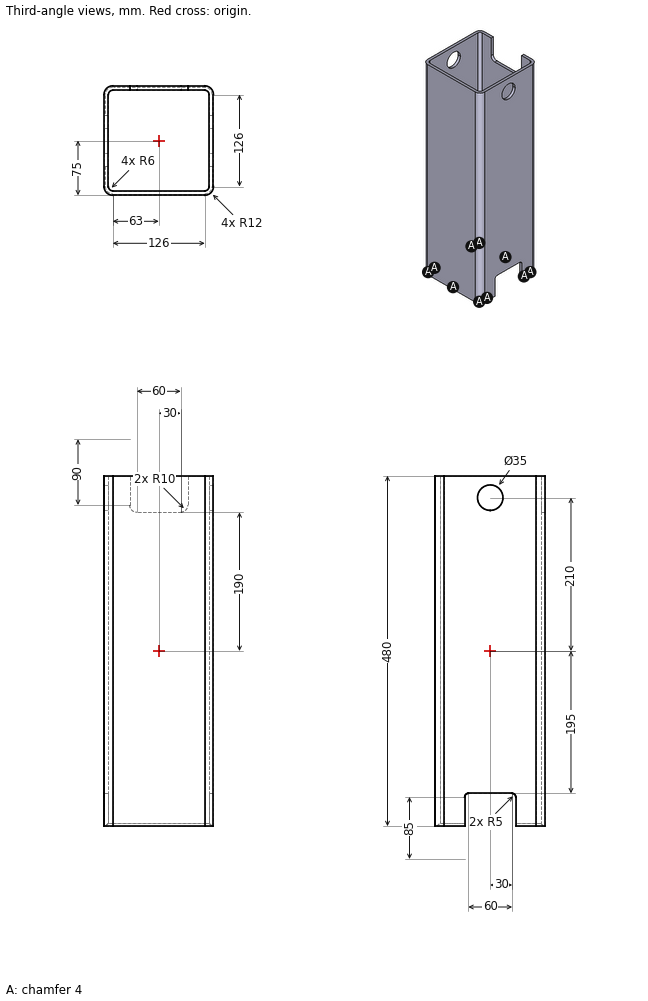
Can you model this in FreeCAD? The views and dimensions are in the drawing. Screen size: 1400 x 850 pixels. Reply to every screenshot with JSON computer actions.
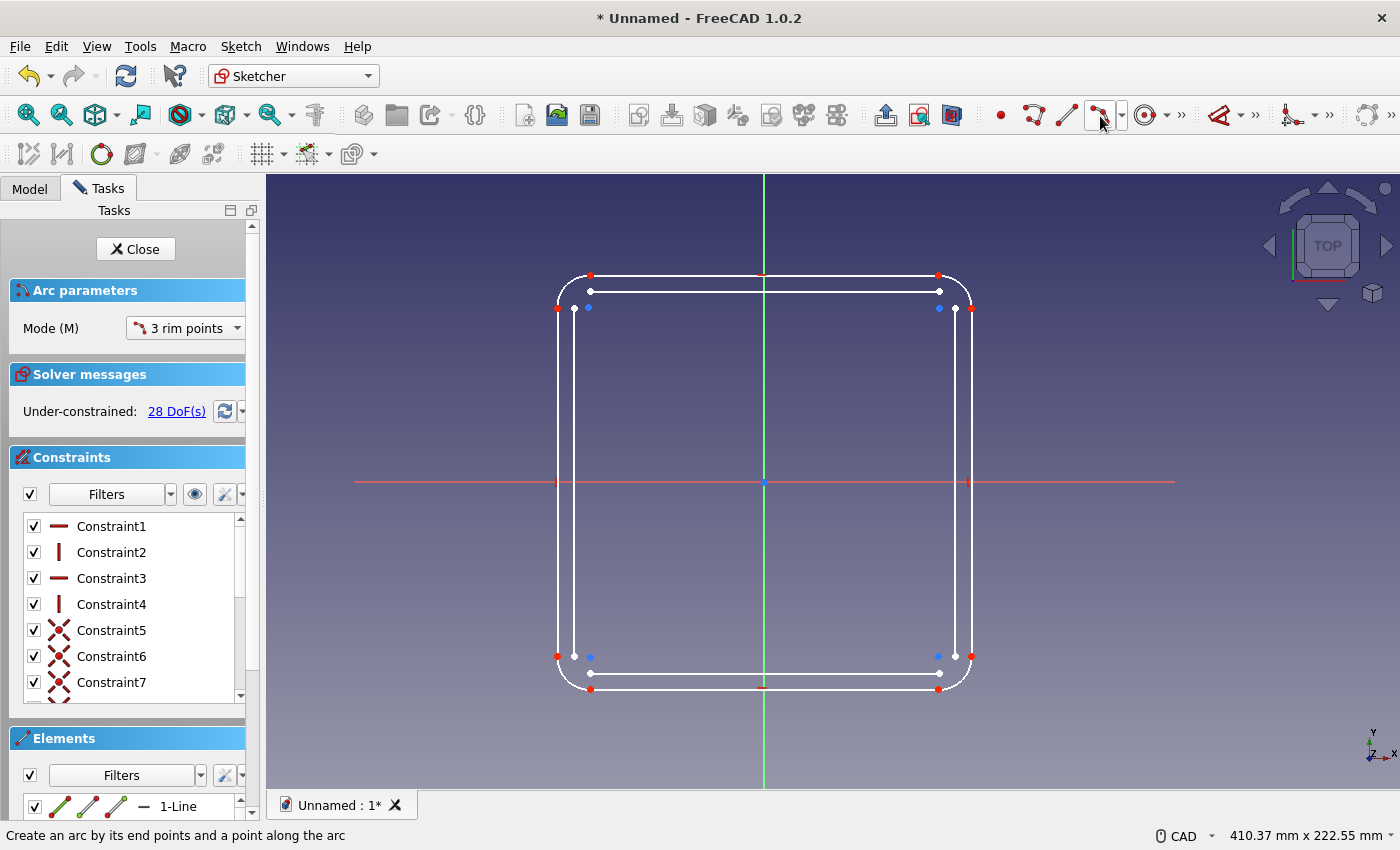
{"action": "left_click", "coordinate": [590, 674]}
{"action": "left_click", "coordinate": [574, 657]}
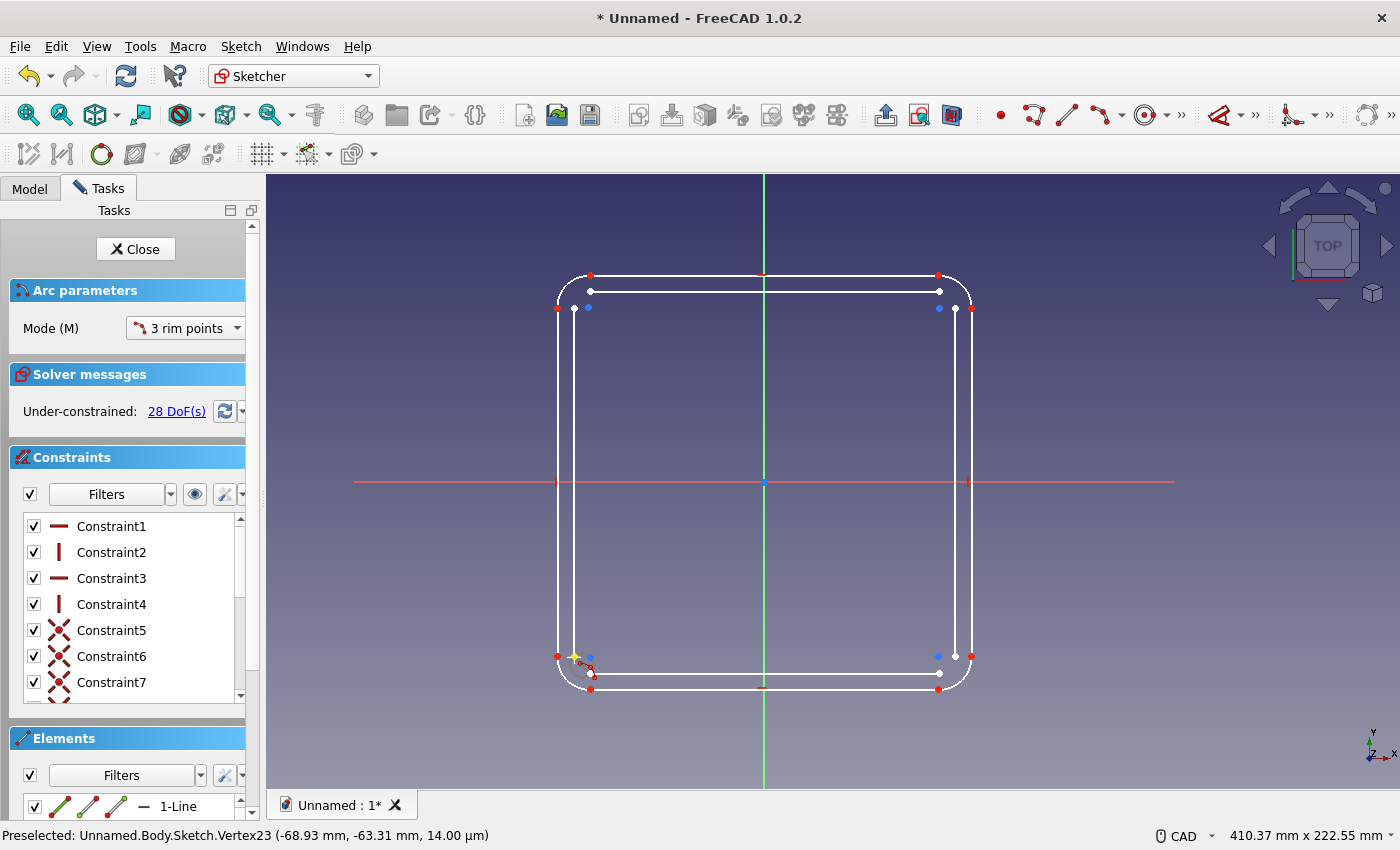
{"action": "scroll", "coordinate": [579, 668], "scroll_direction": "up", "scroll_amount": 6}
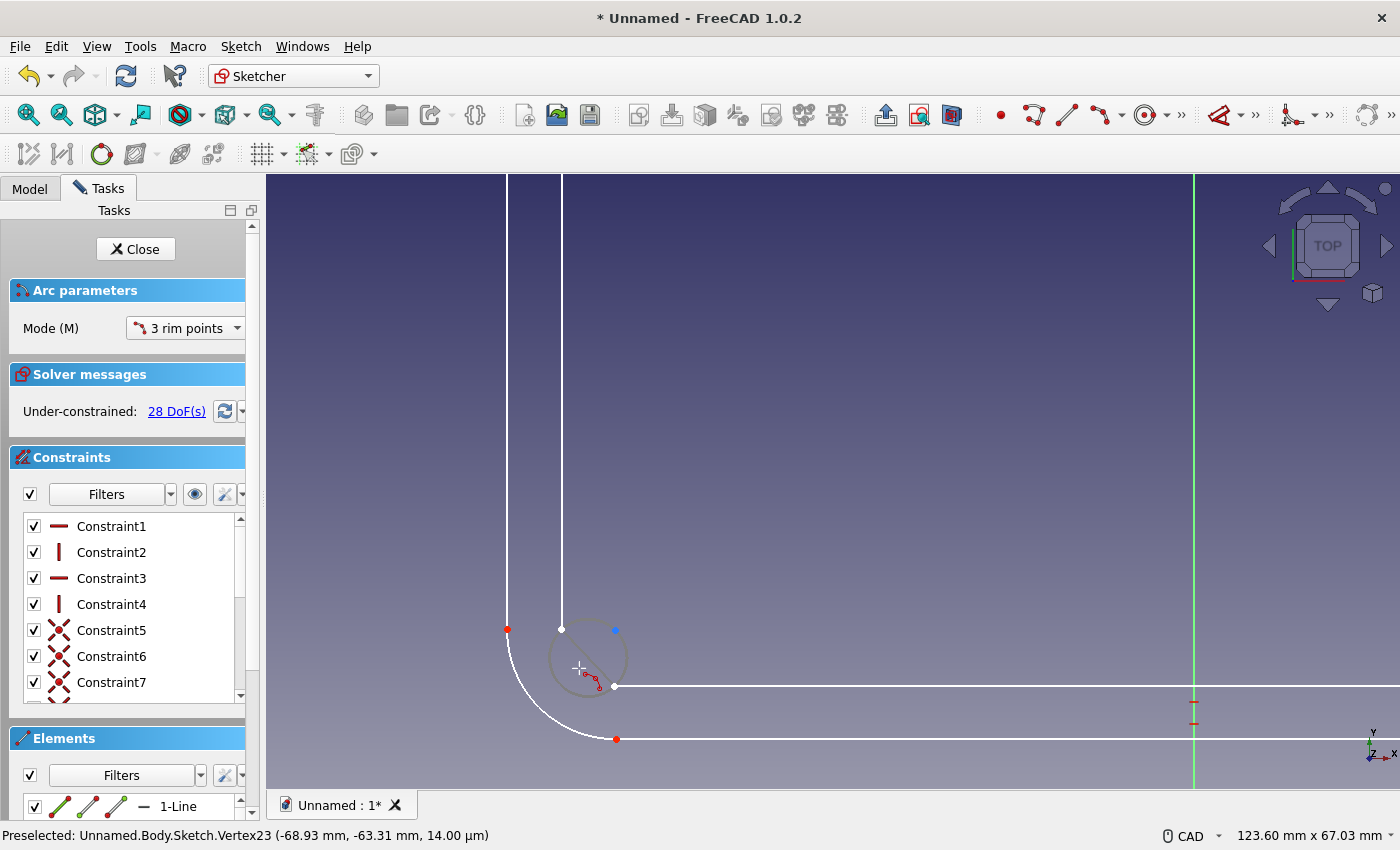
{"action": "left_click", "coordinate": [577, 666]}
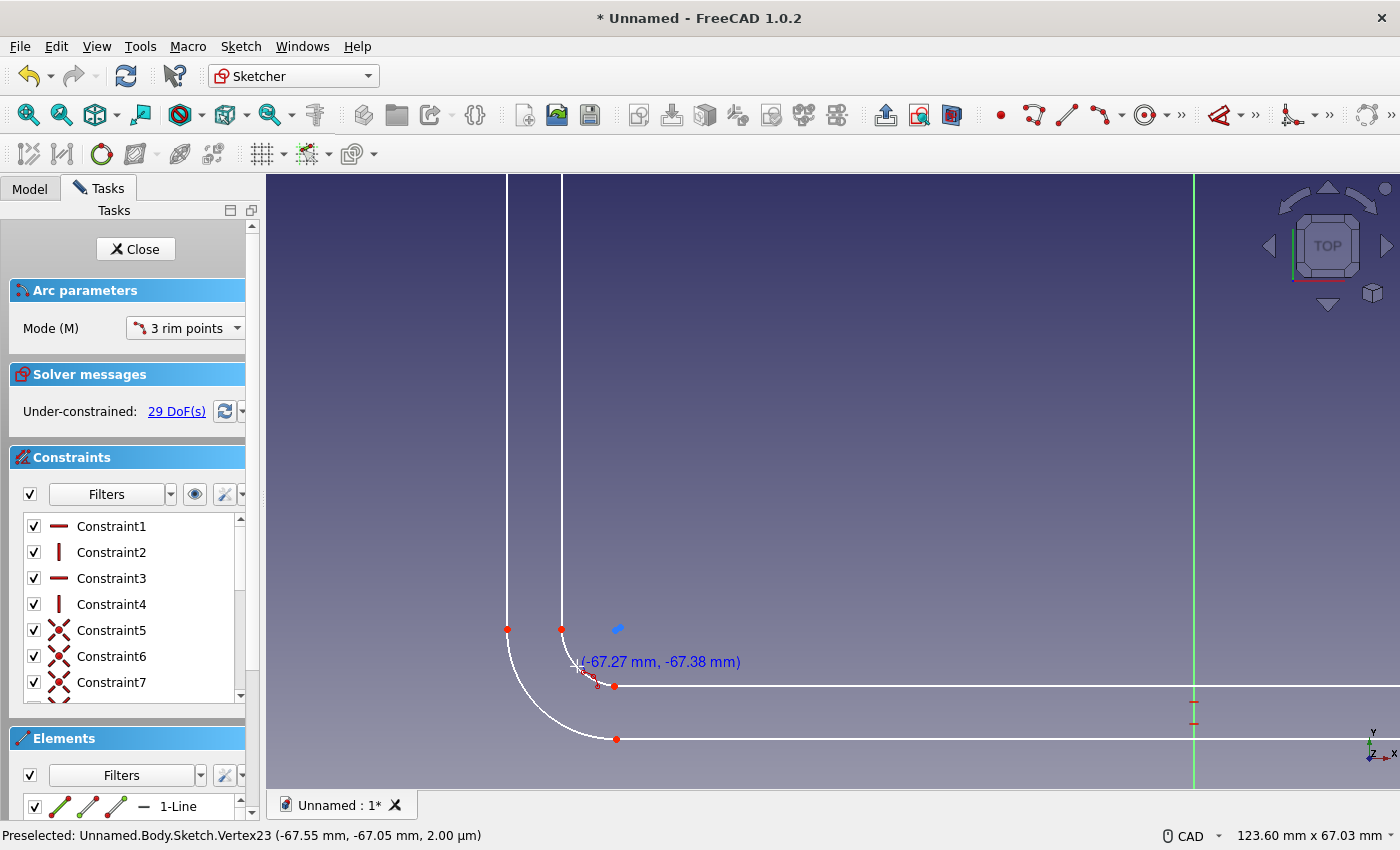
{"action": "scroll", "coordinate": [579, 668], "scroll_direction": "down", "scroll_amount": 6}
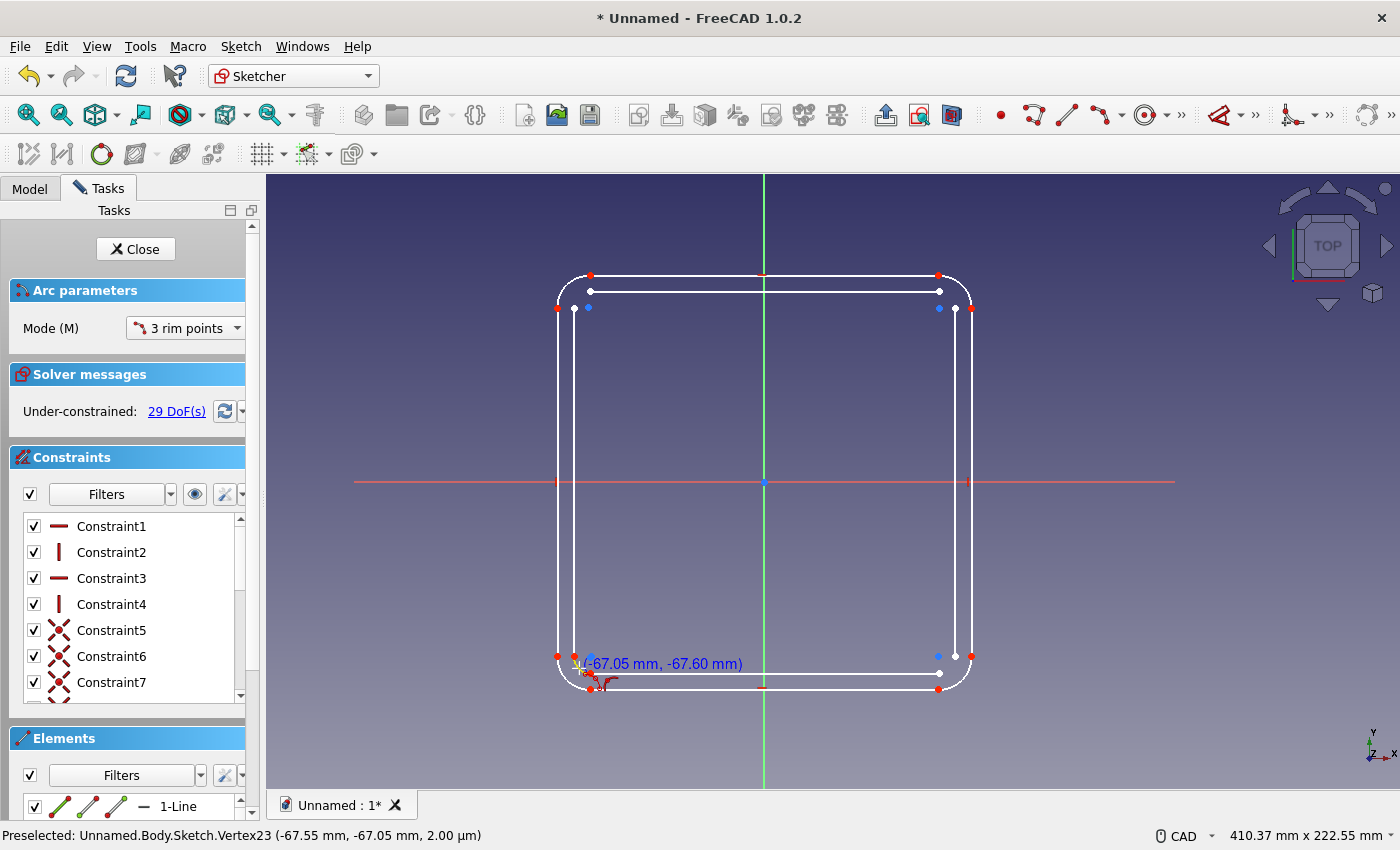
{"action": "left_click", "coordinate": [574, 309]}
{"action": "left_click", "coordinate": [590, 292]}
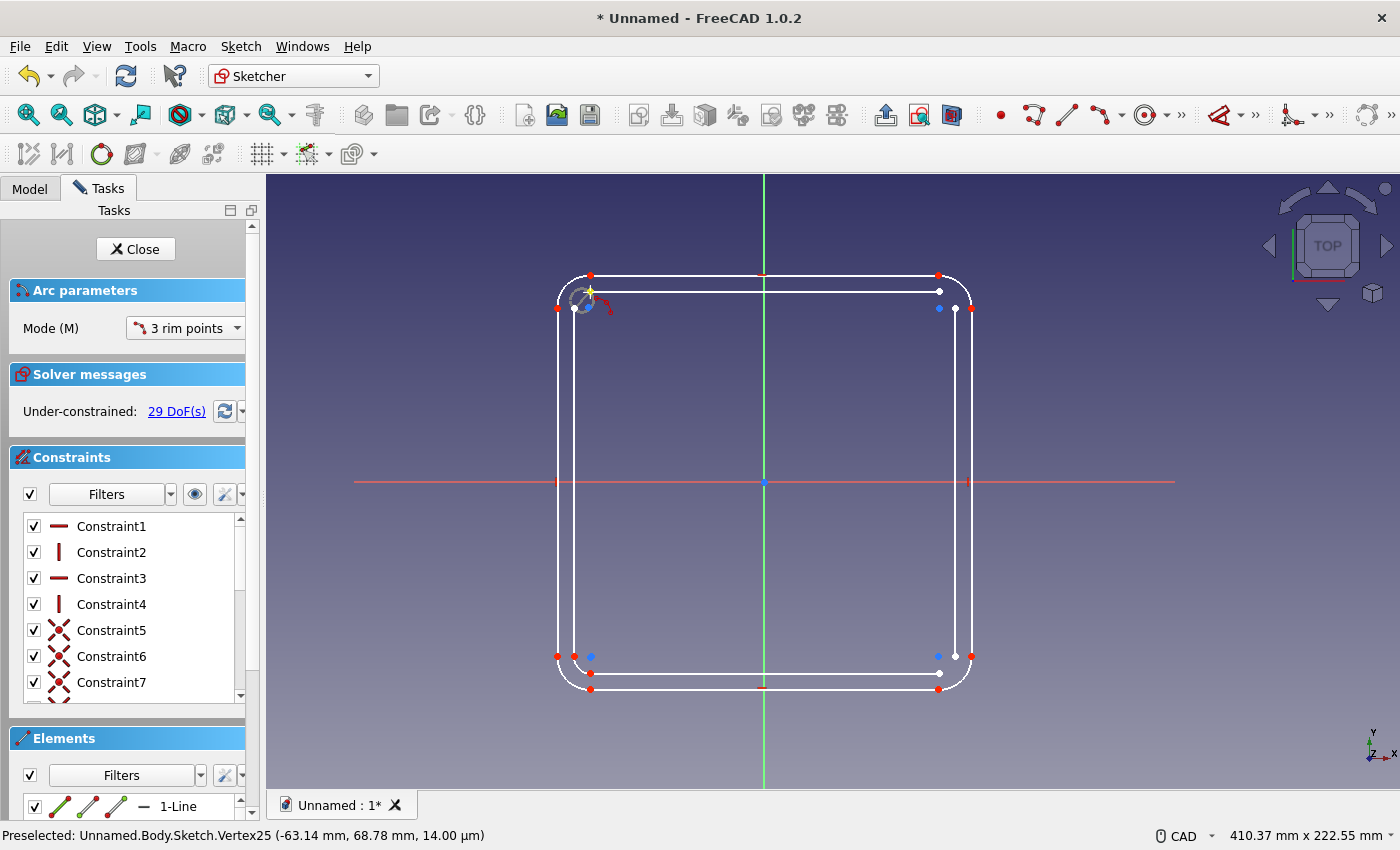
{"action": "scroll", "coordinate": [579, 296], "scroll_direction": "up", "scroll_amount": 6}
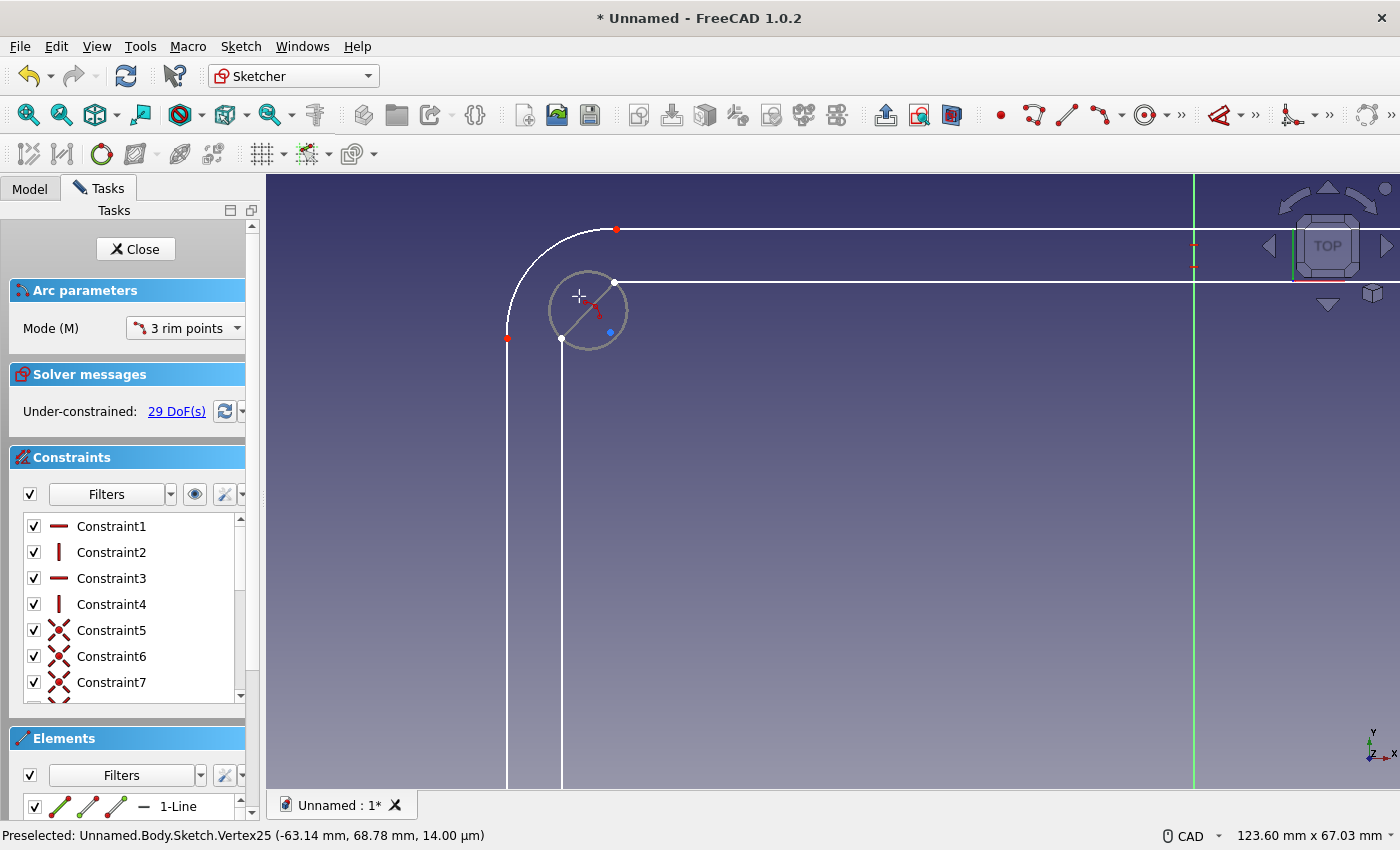
{"action": "left_click", "coordinate": [577, 296]}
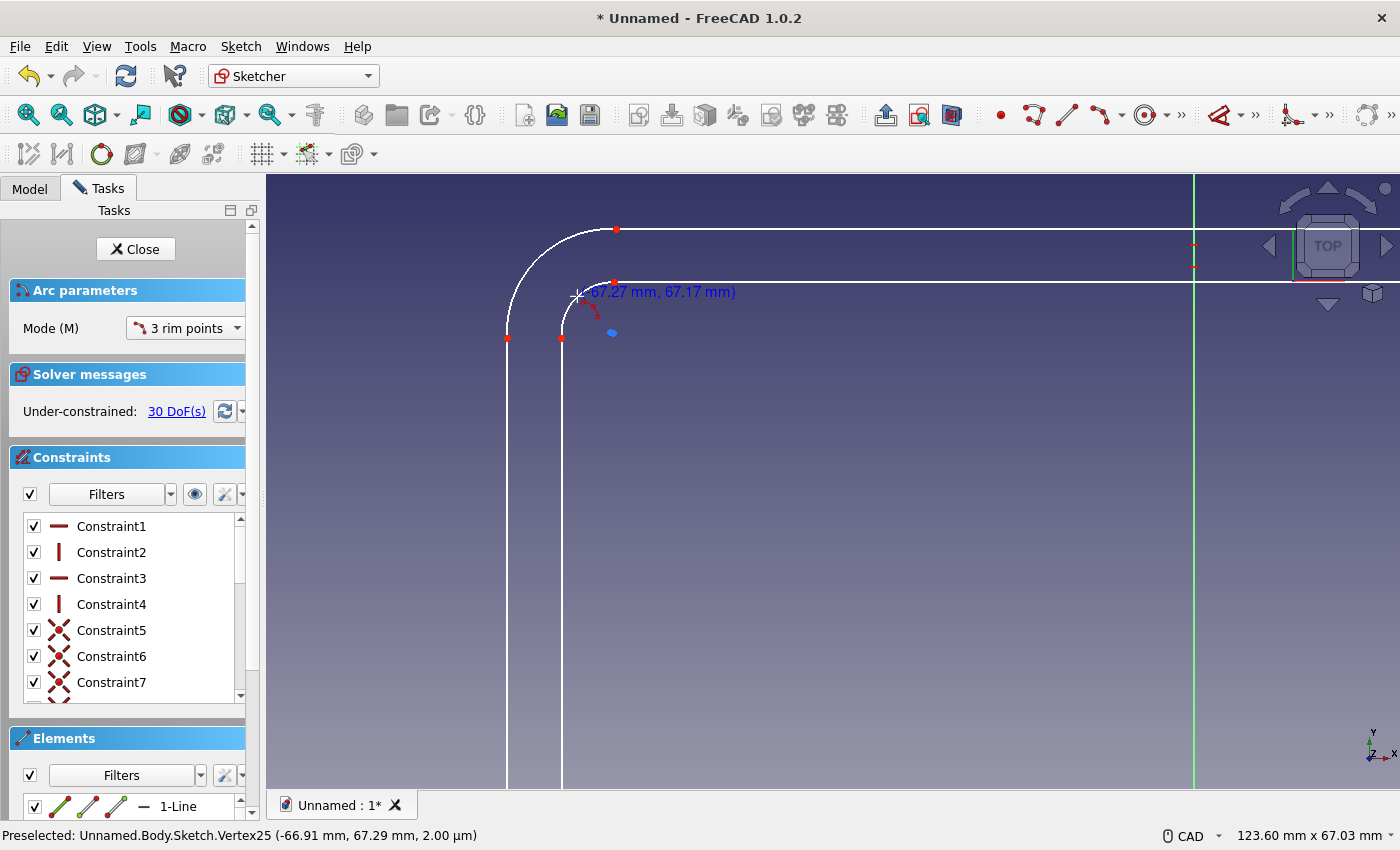
{"action": "scroll", "coordinate": [579, 295], "scroll_direction": "down", "scroll_amount": 6}